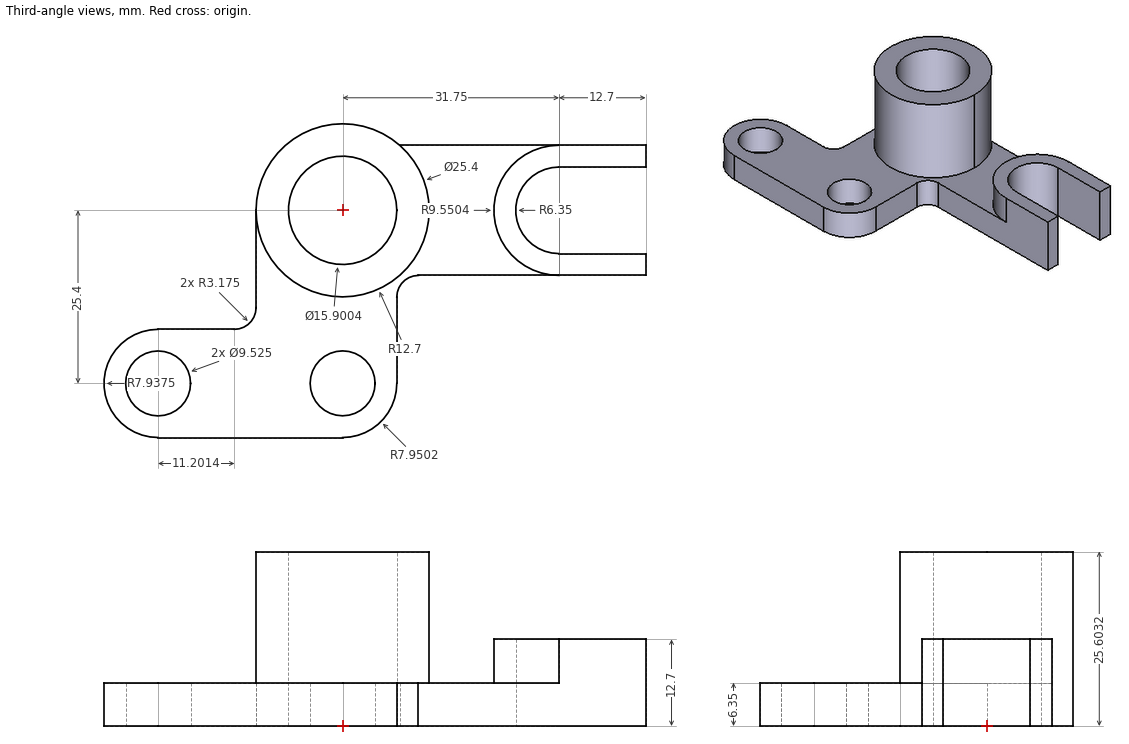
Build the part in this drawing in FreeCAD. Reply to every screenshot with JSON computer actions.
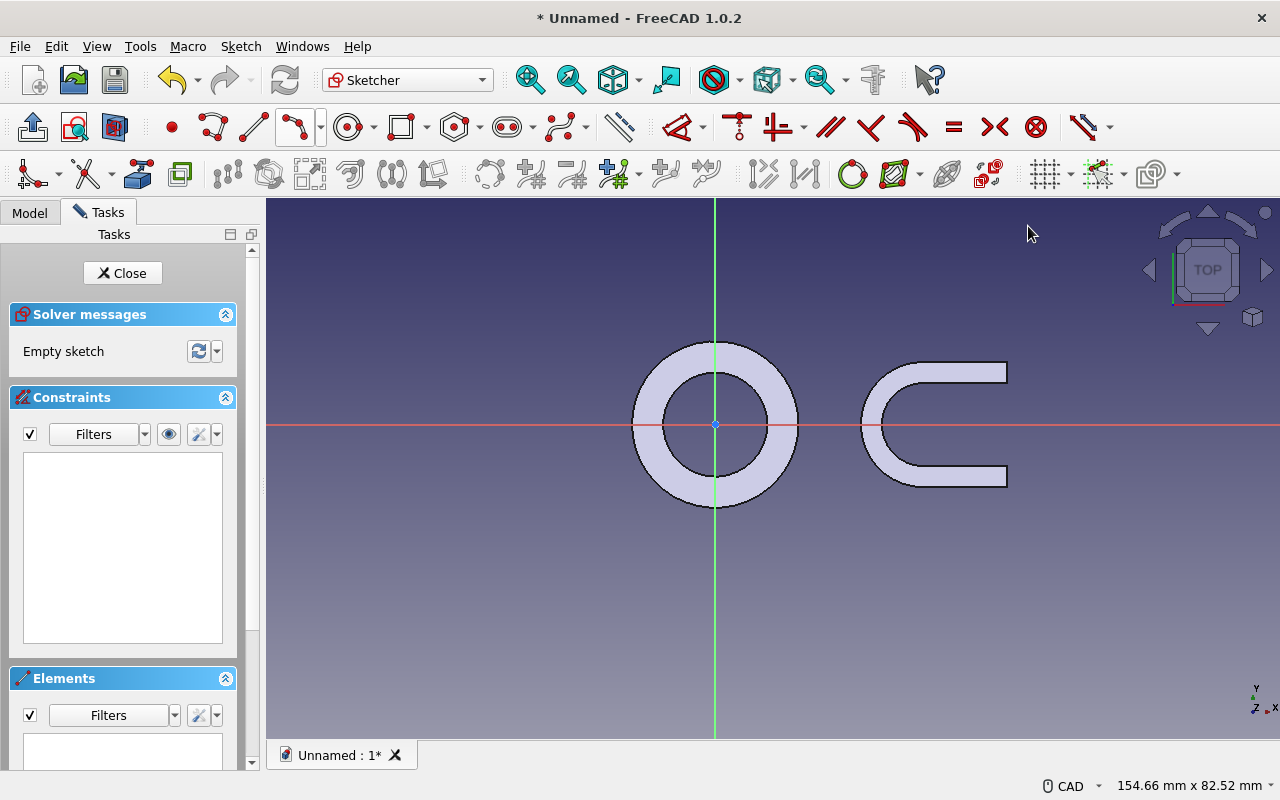
{"action": "left_click", "coordinate": [254, 128]}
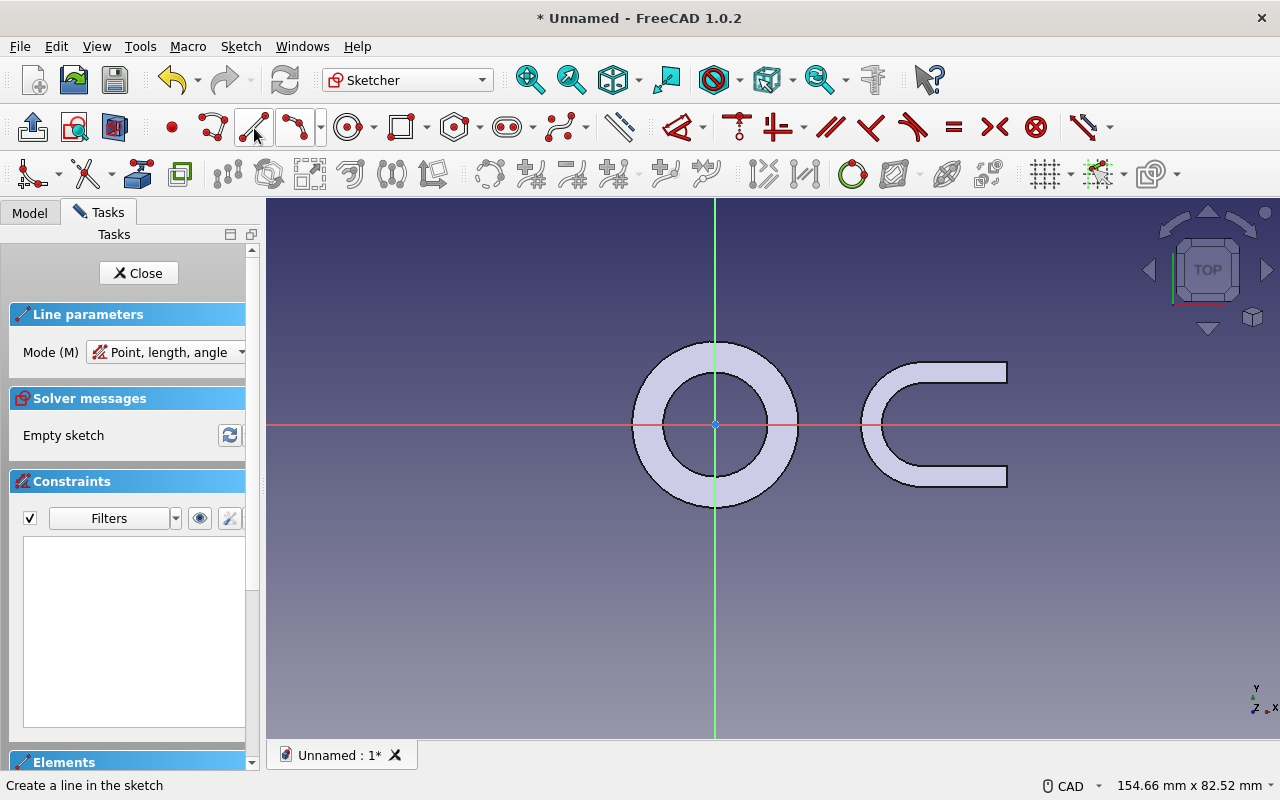
{"action": "left_click", "coordinate": [632, 425]}
{"action": "left_click", "coordinate": [632, 518]}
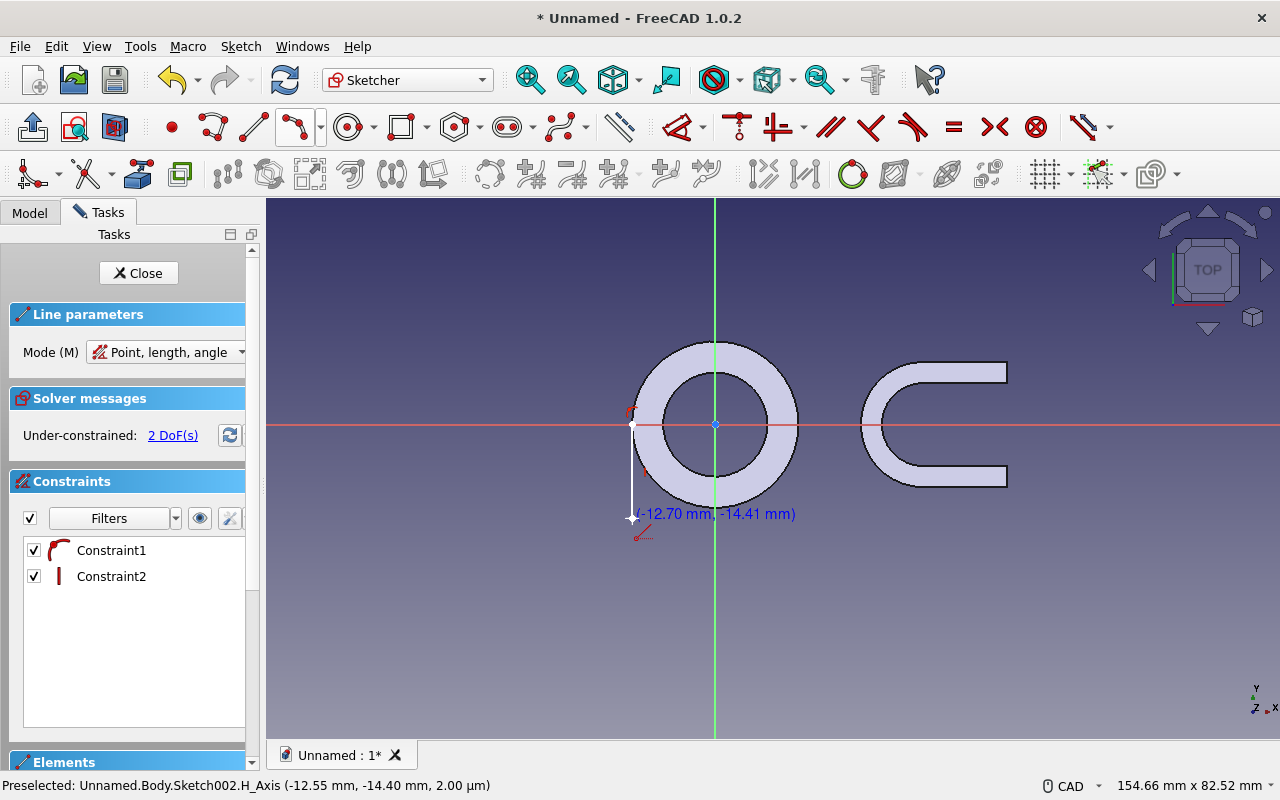
{"action": "left_click", "coordinate": [611, 539]}
{"action": "left_click", "coordinate": [538, 539]}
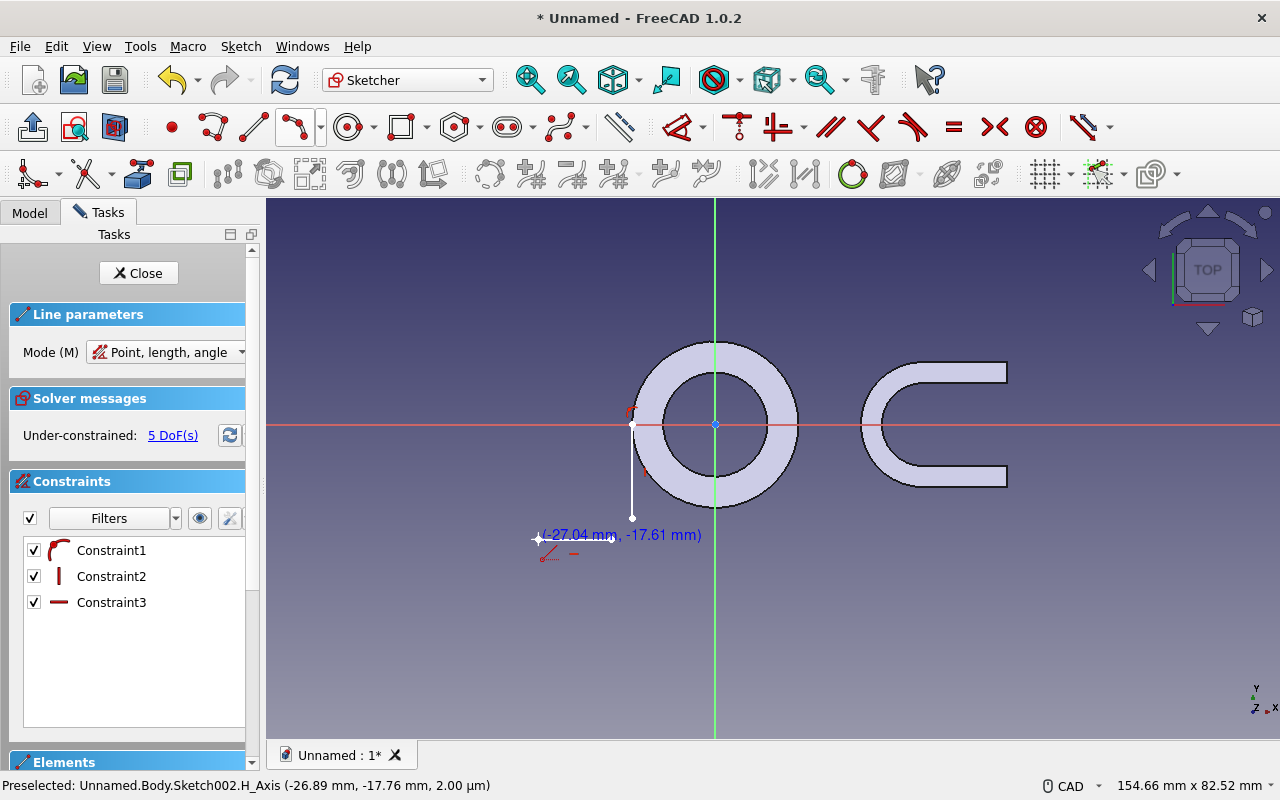
{"action": "left_click", "coordinate": [538, 643]}
{"action": "left_click", "coordinate": [715, 643]}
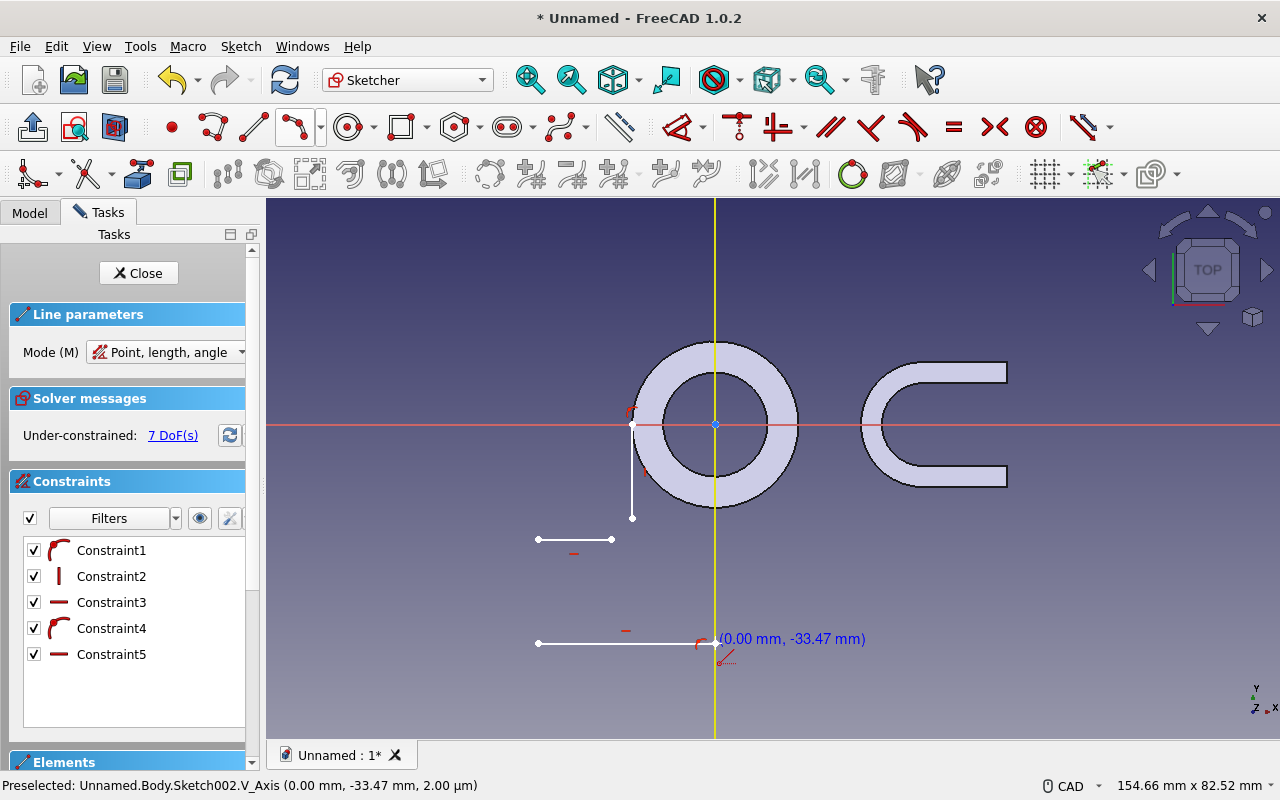
{"action": "left_click", "coordinate": [767, 591]}
{"action": "left_click", "coordinate": [767, 508]}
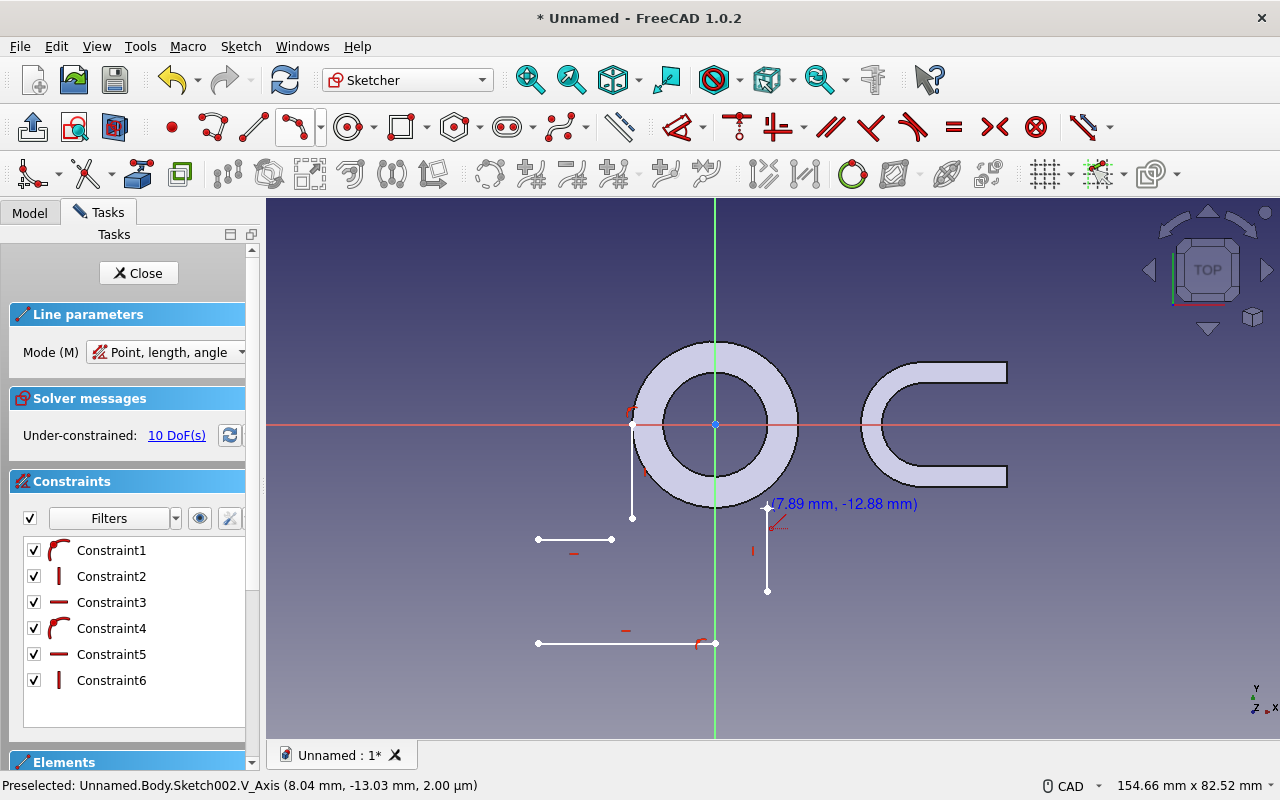
{"action": "left_click", "coordinate": [788, 487]}
{"action": "left_click", "coordinate": [923, 487]}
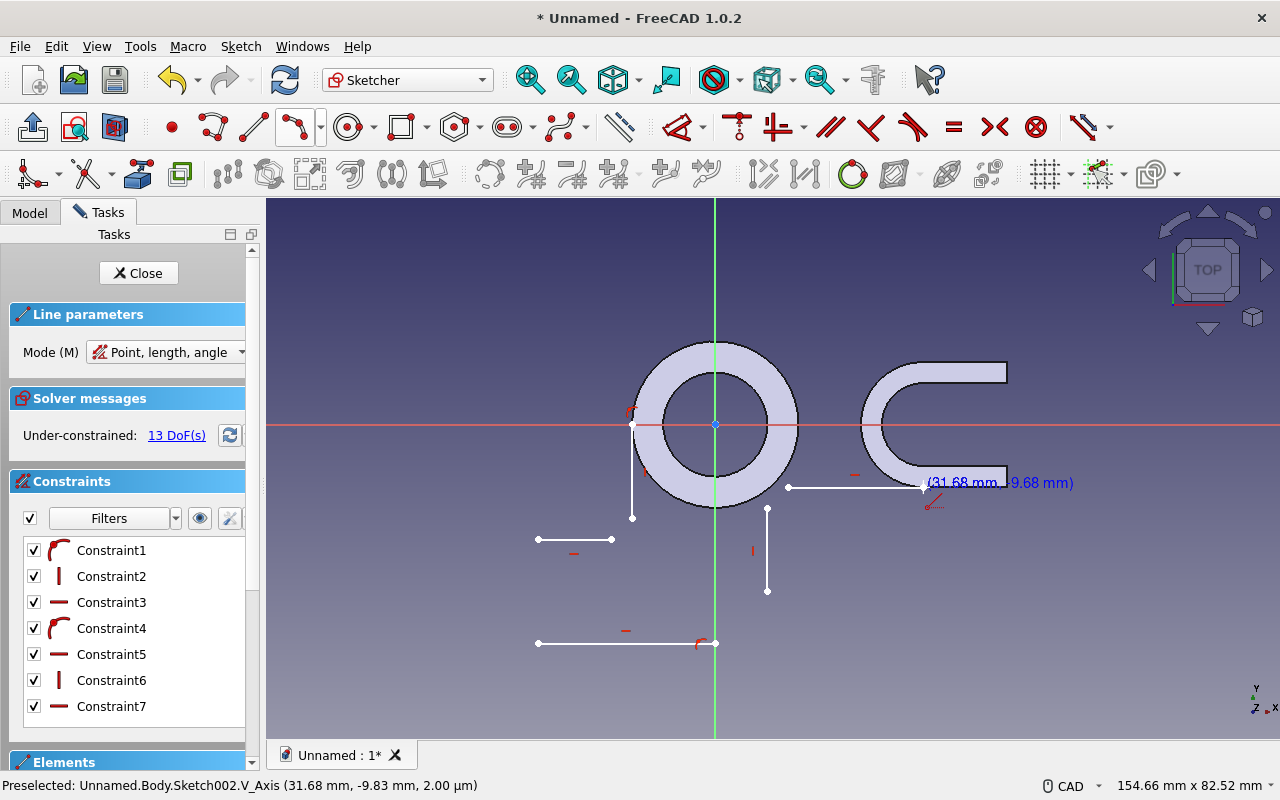
{"action": "left_click", "coordinate": [923, 362]}
{"action": "left_click", "coordinate": [770, 362]}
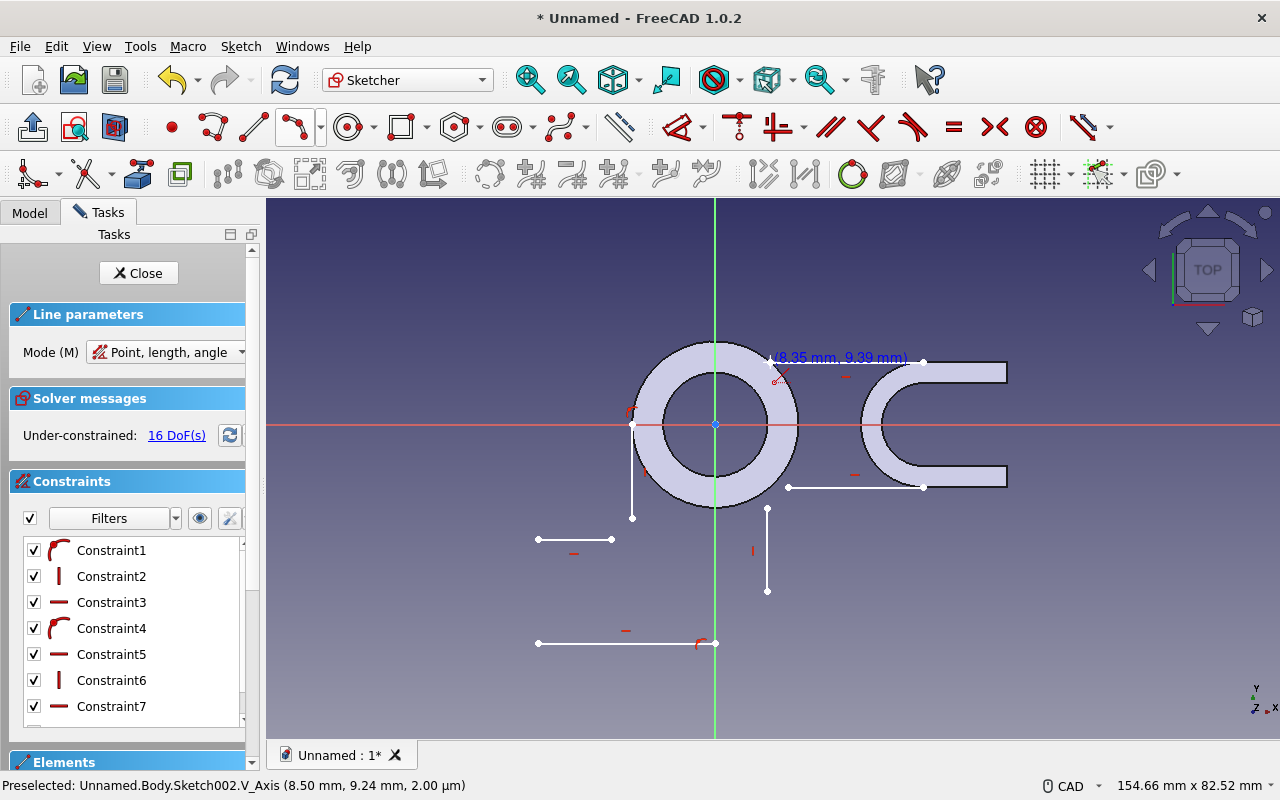
{"action": "left_click", "coordinate": [294, 128]}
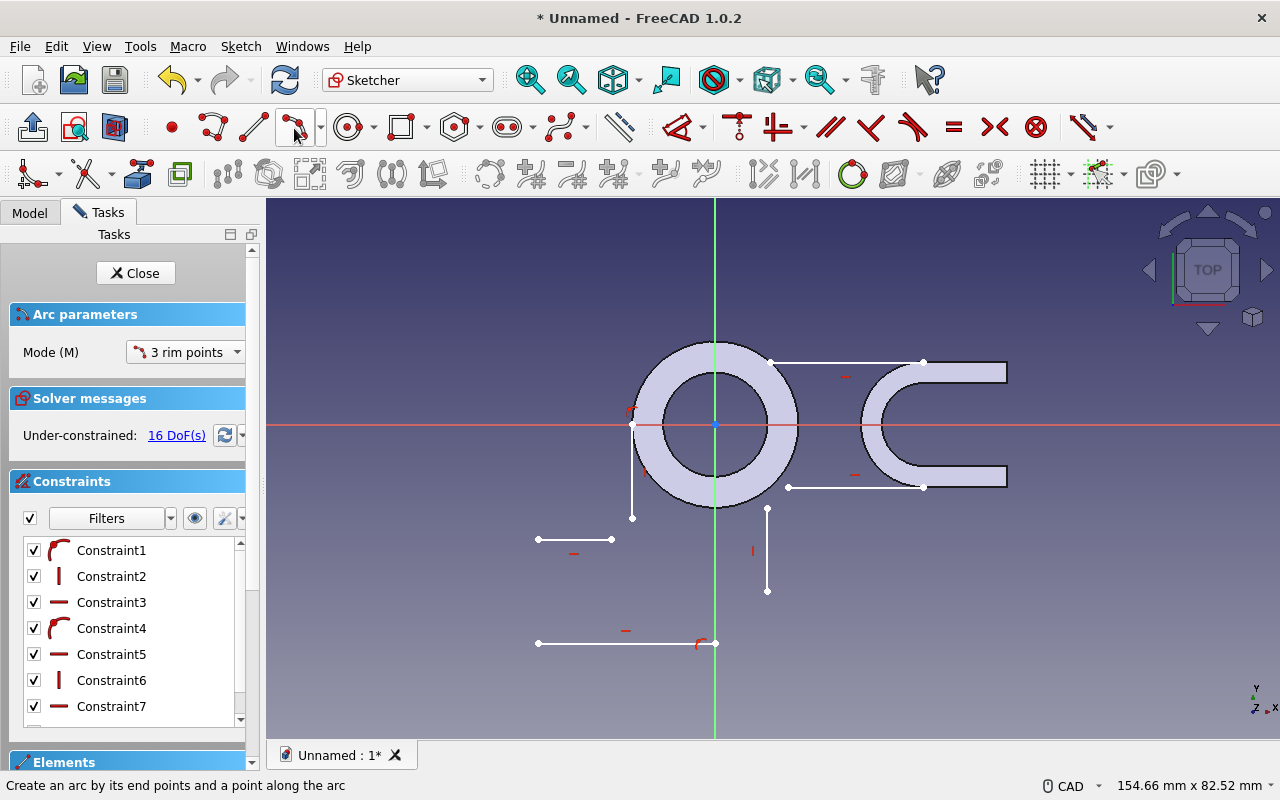
{"action": "left_click", "coordinate": [632, 519]}
{"action": "left_click", "coordinate": [611, 540]}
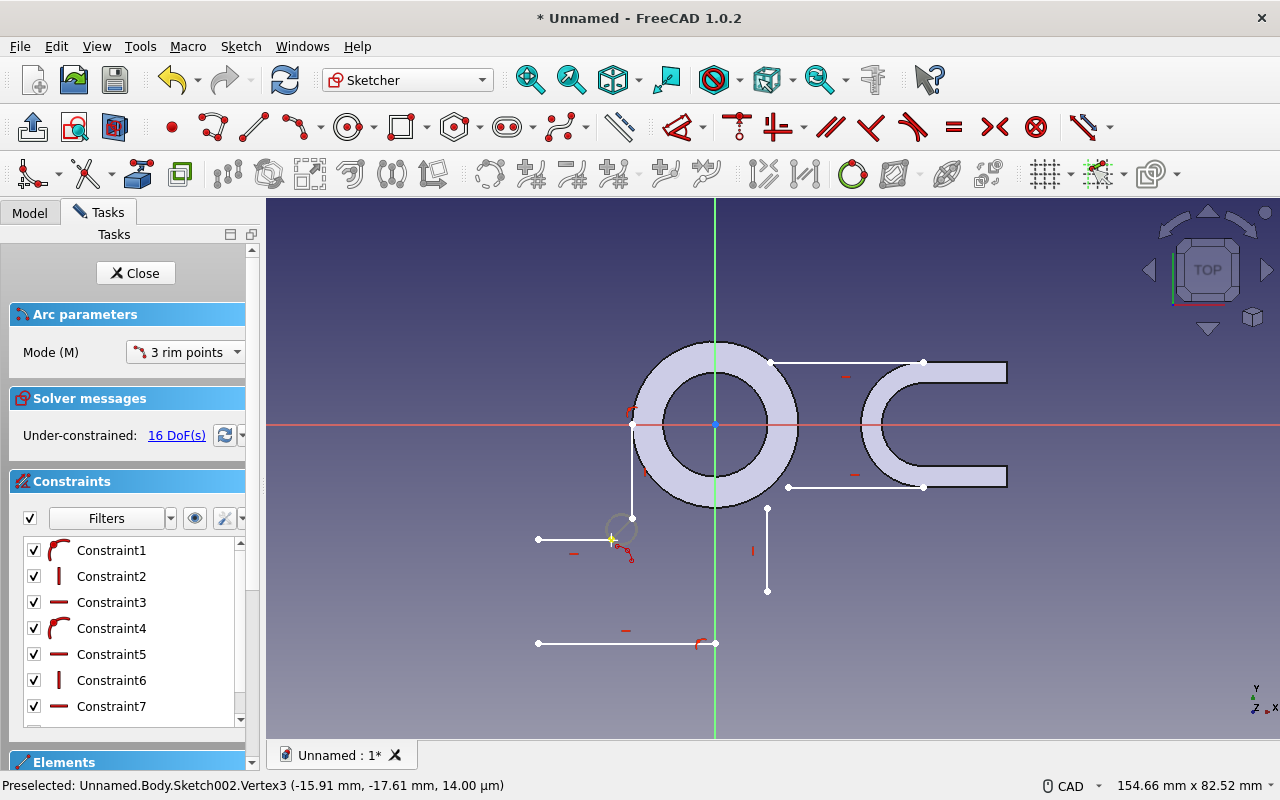
{"action": "scroll", "coordinate": [626, 533], "scroll_direction": "up", "scroll_amount": 5}